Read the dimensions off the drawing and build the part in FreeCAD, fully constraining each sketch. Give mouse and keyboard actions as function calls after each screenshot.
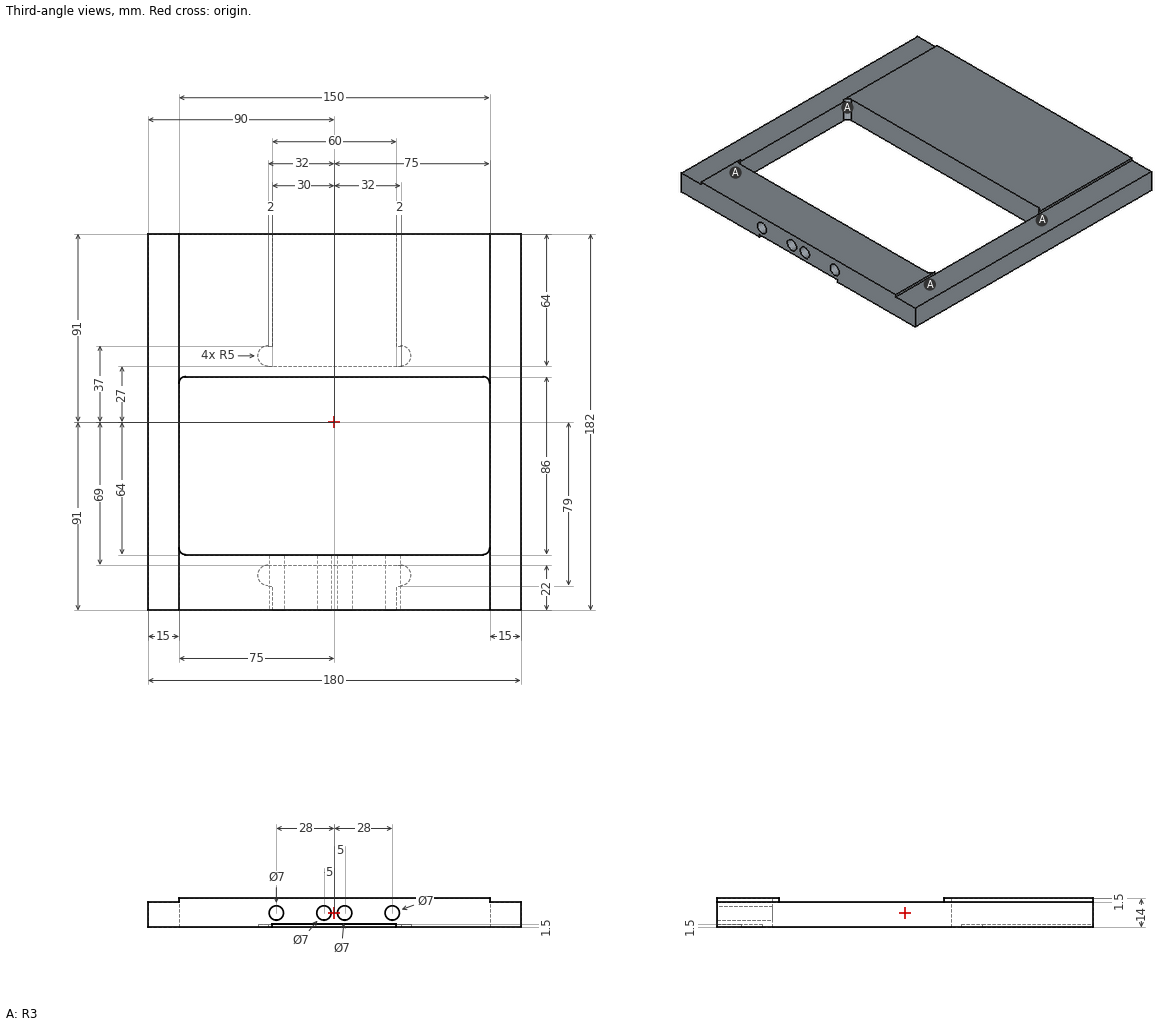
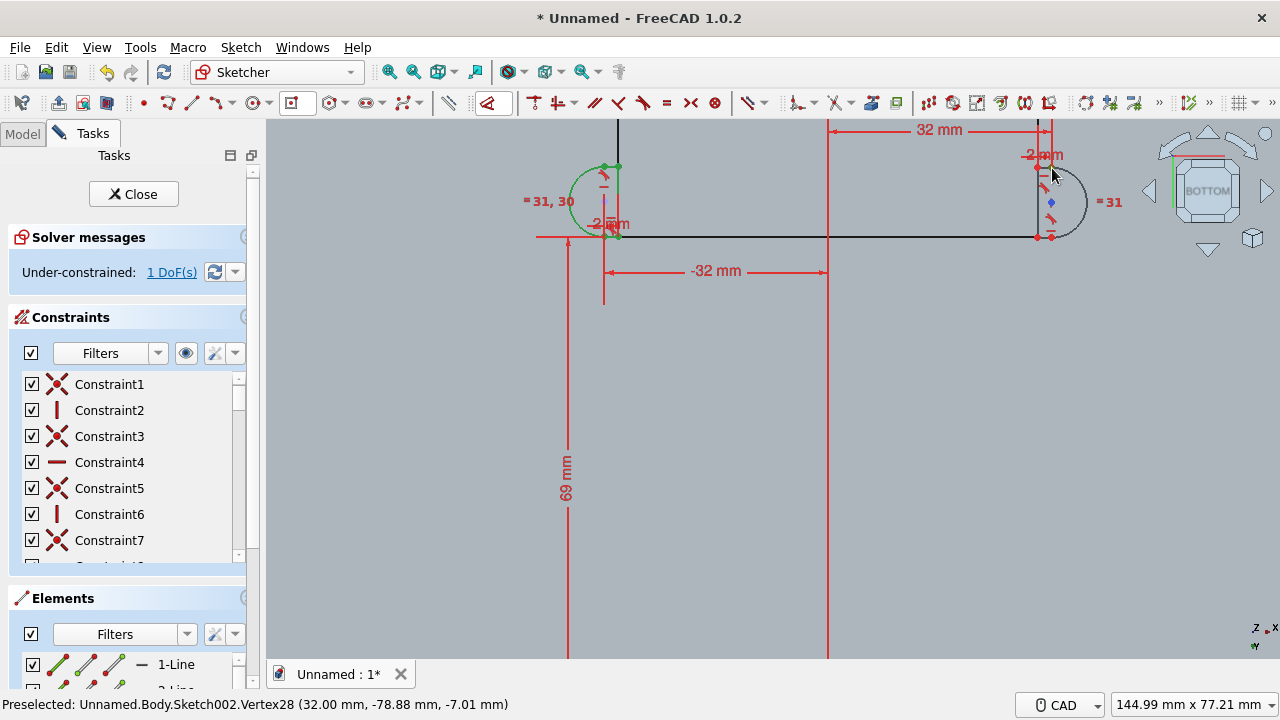
key(i)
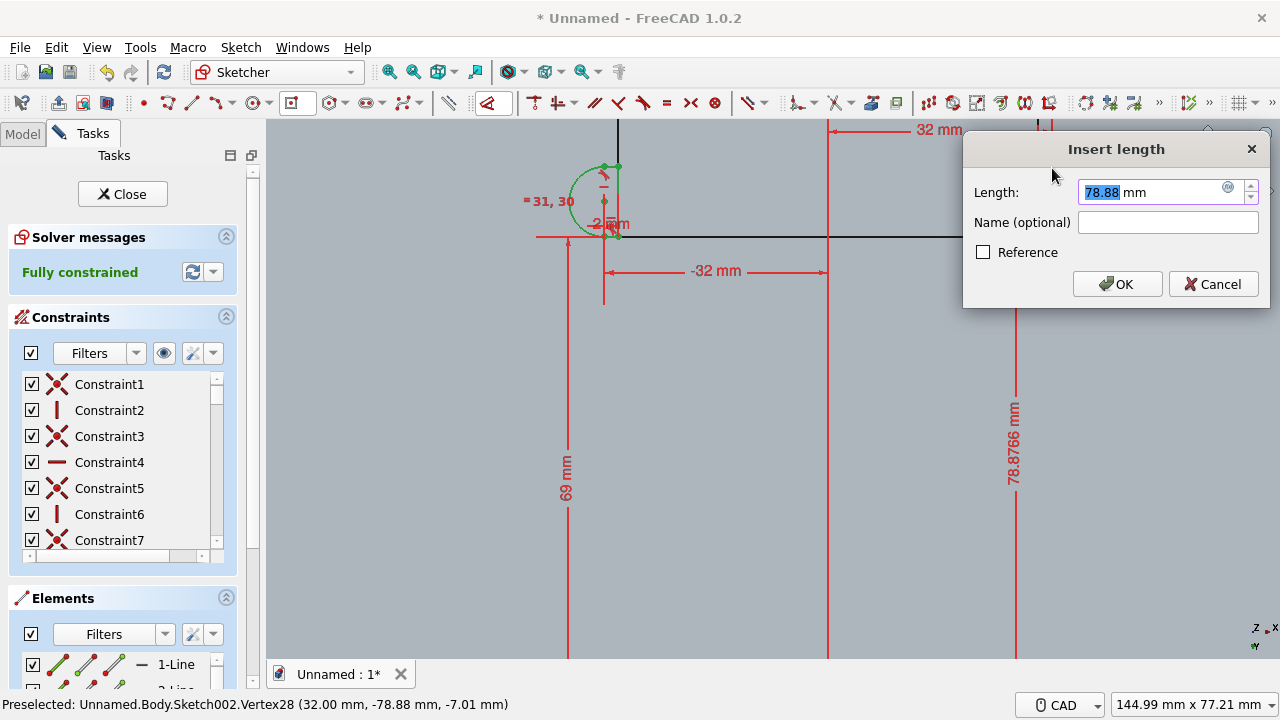
text(79)
key(Return)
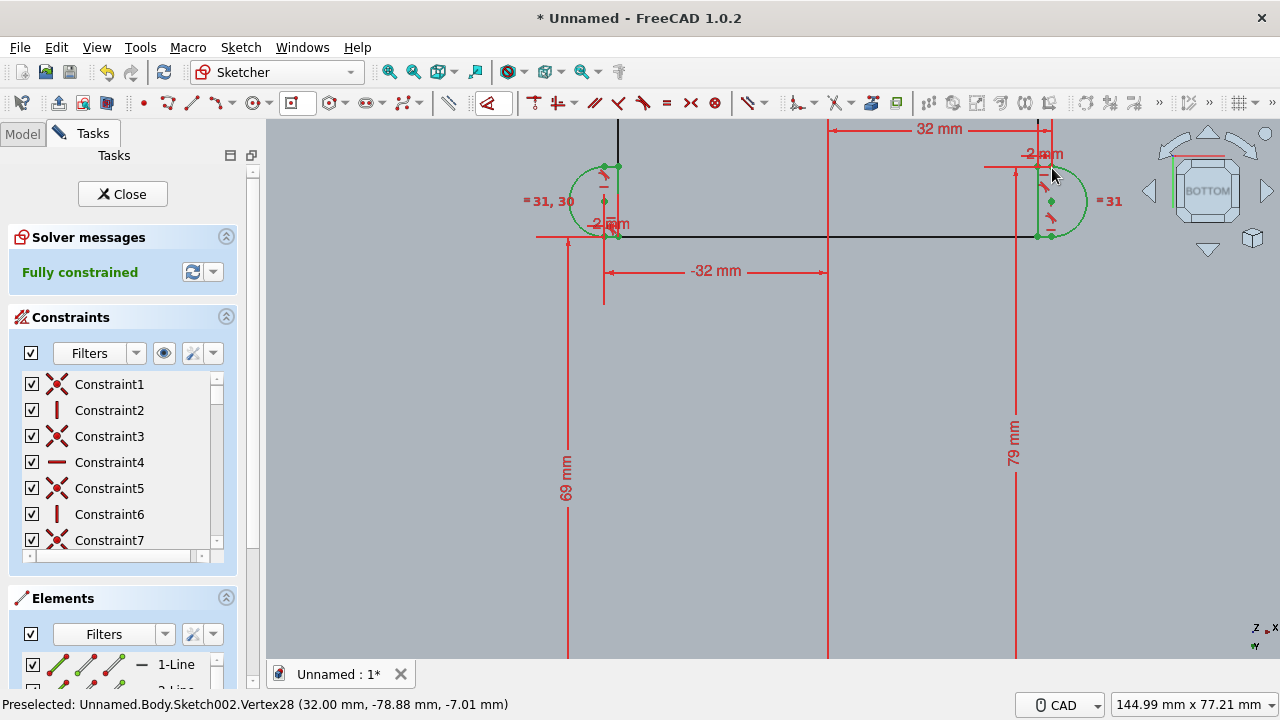
click(123, 194)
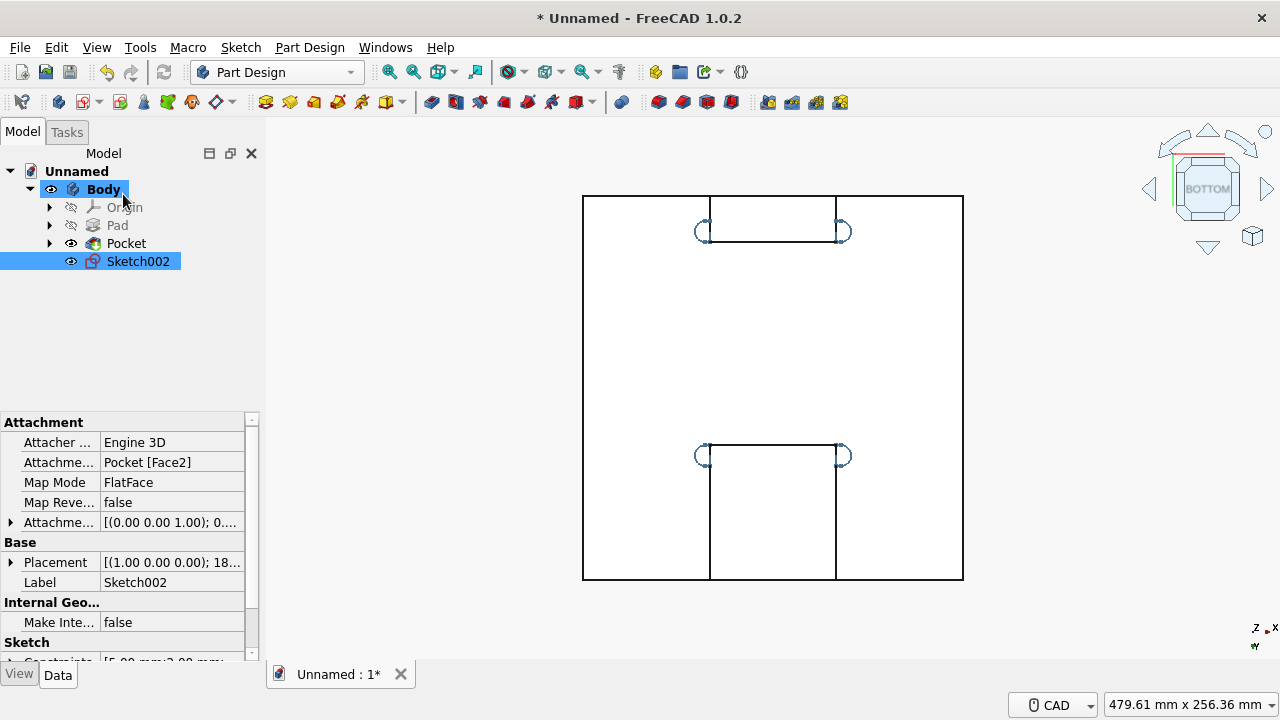
click(432, 102)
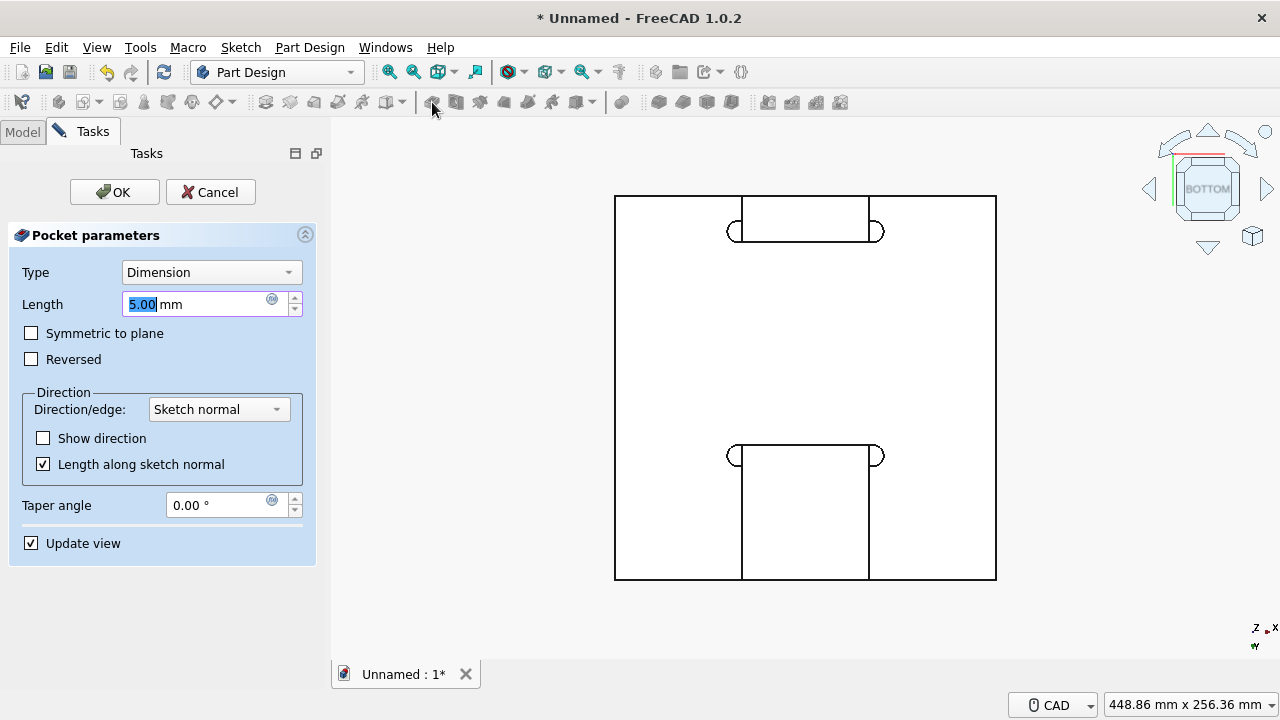
text(1.5)
key(Tab)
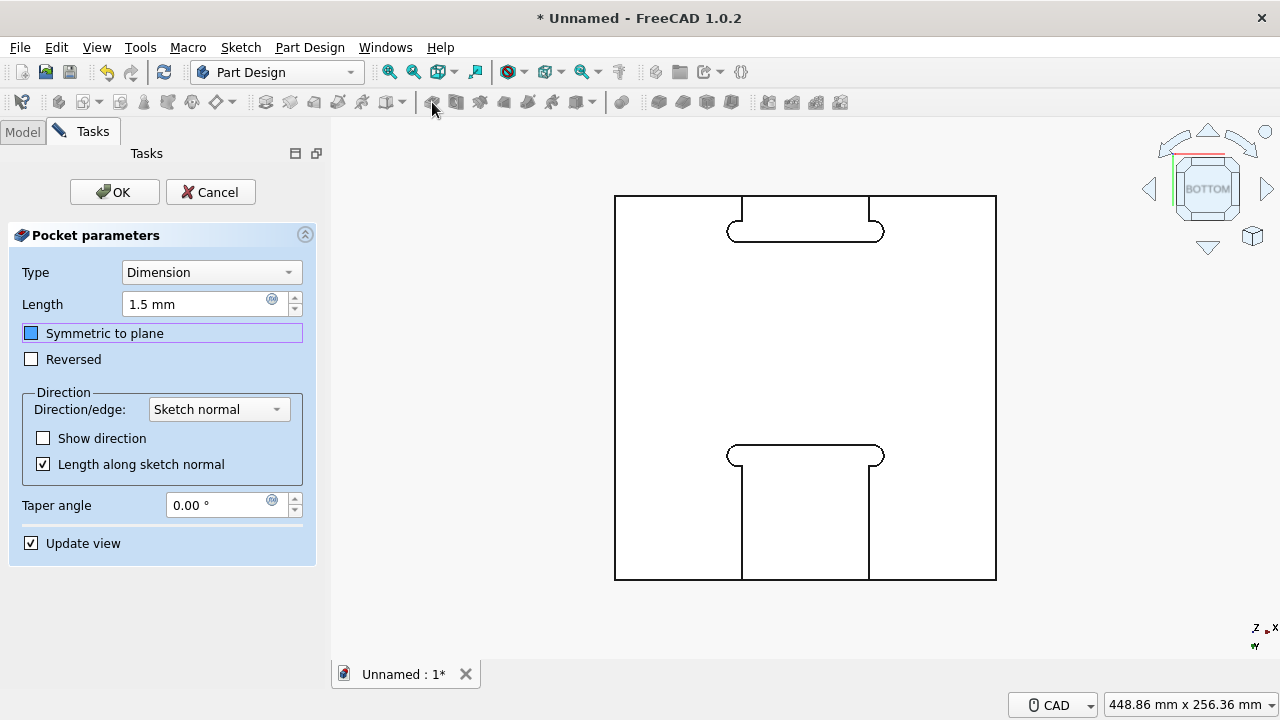
click(115, 192)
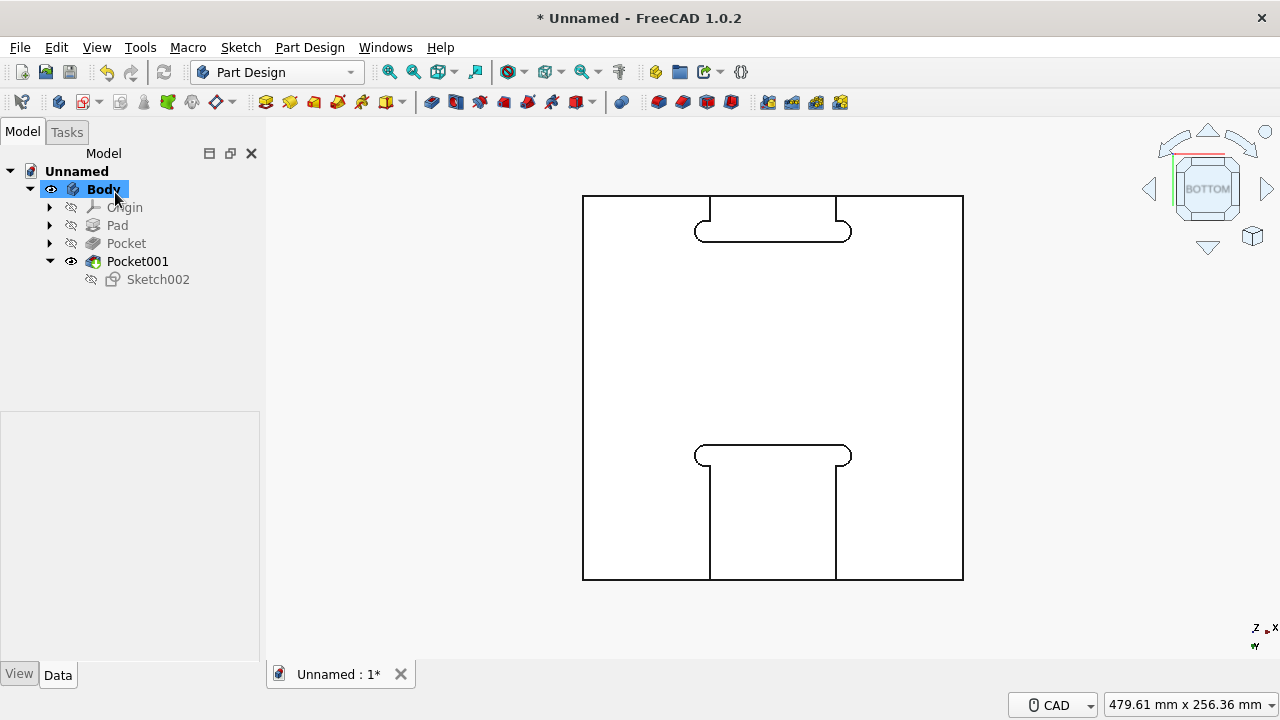
click(827, 332)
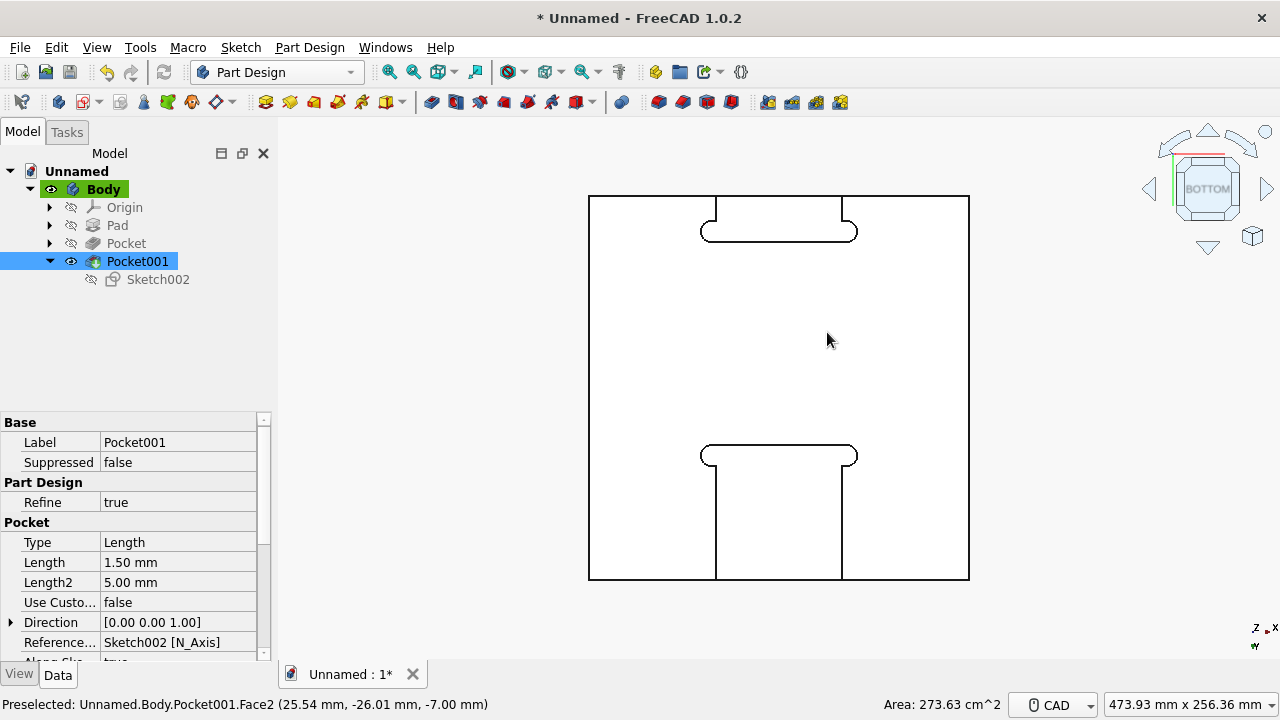
click(84, 102)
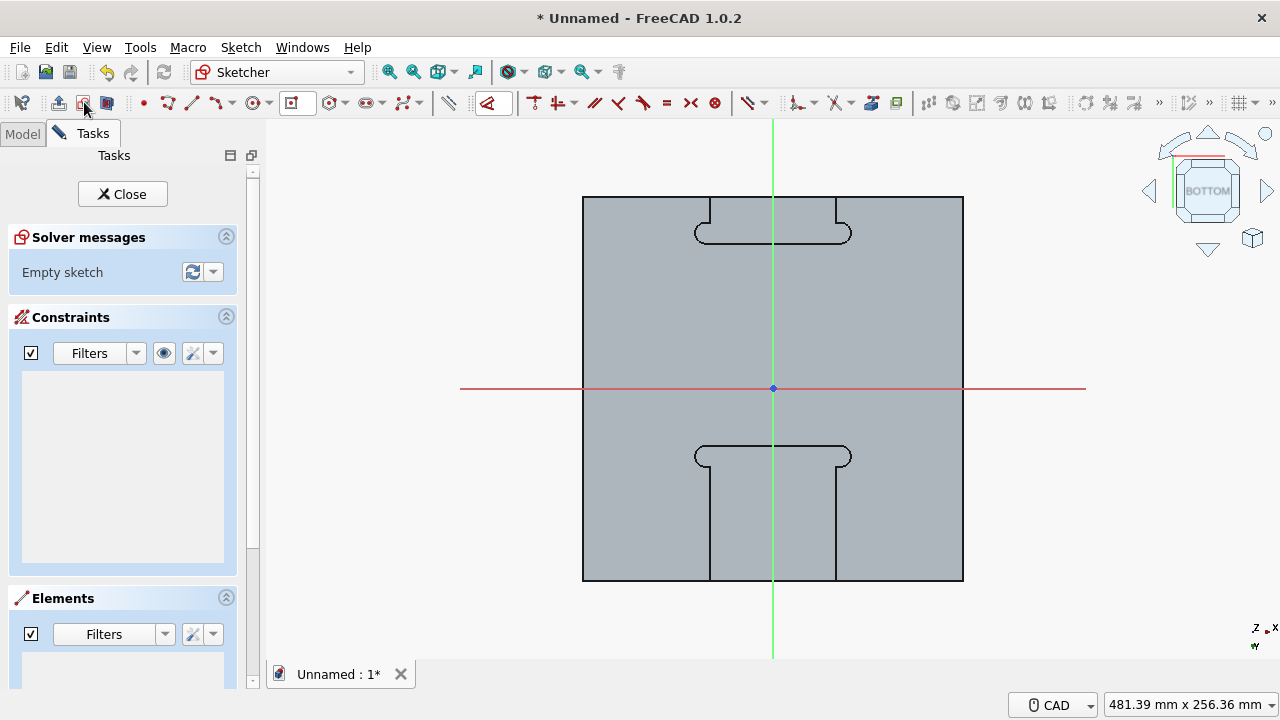
scroll(856, 291, up, 3)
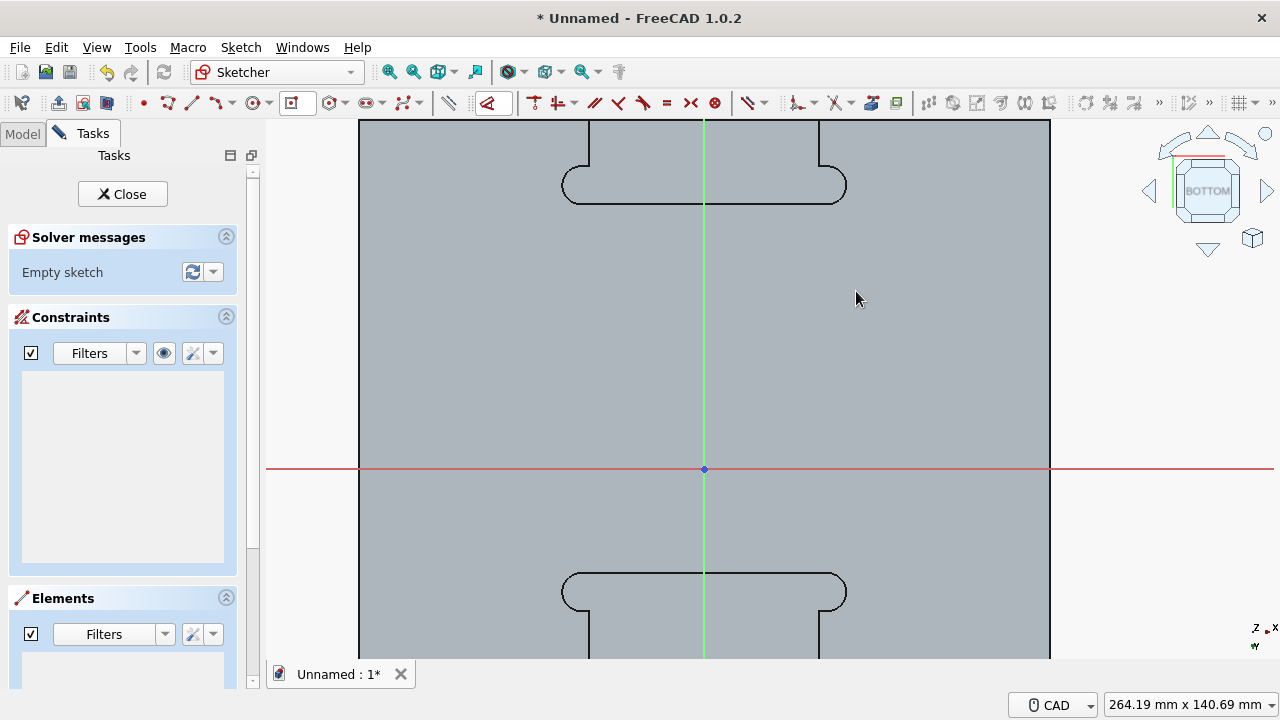
key(g)
key(r)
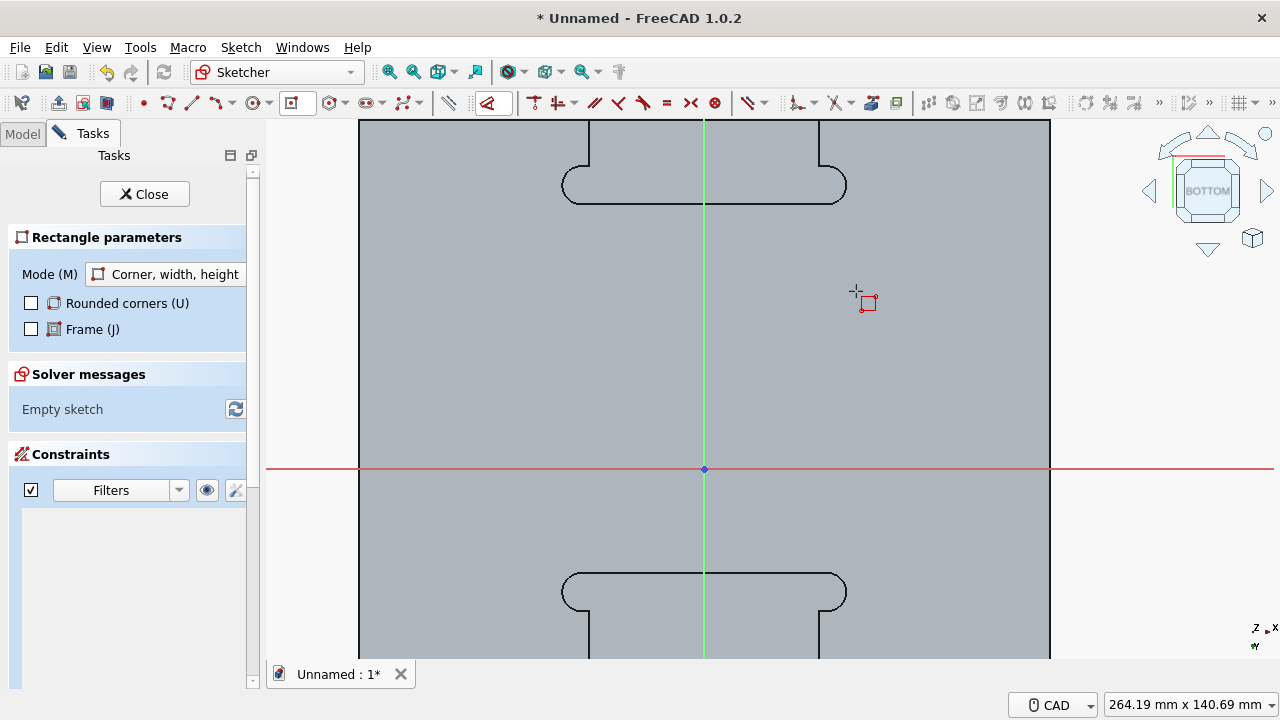
click(416, 224)
move(992, 554)